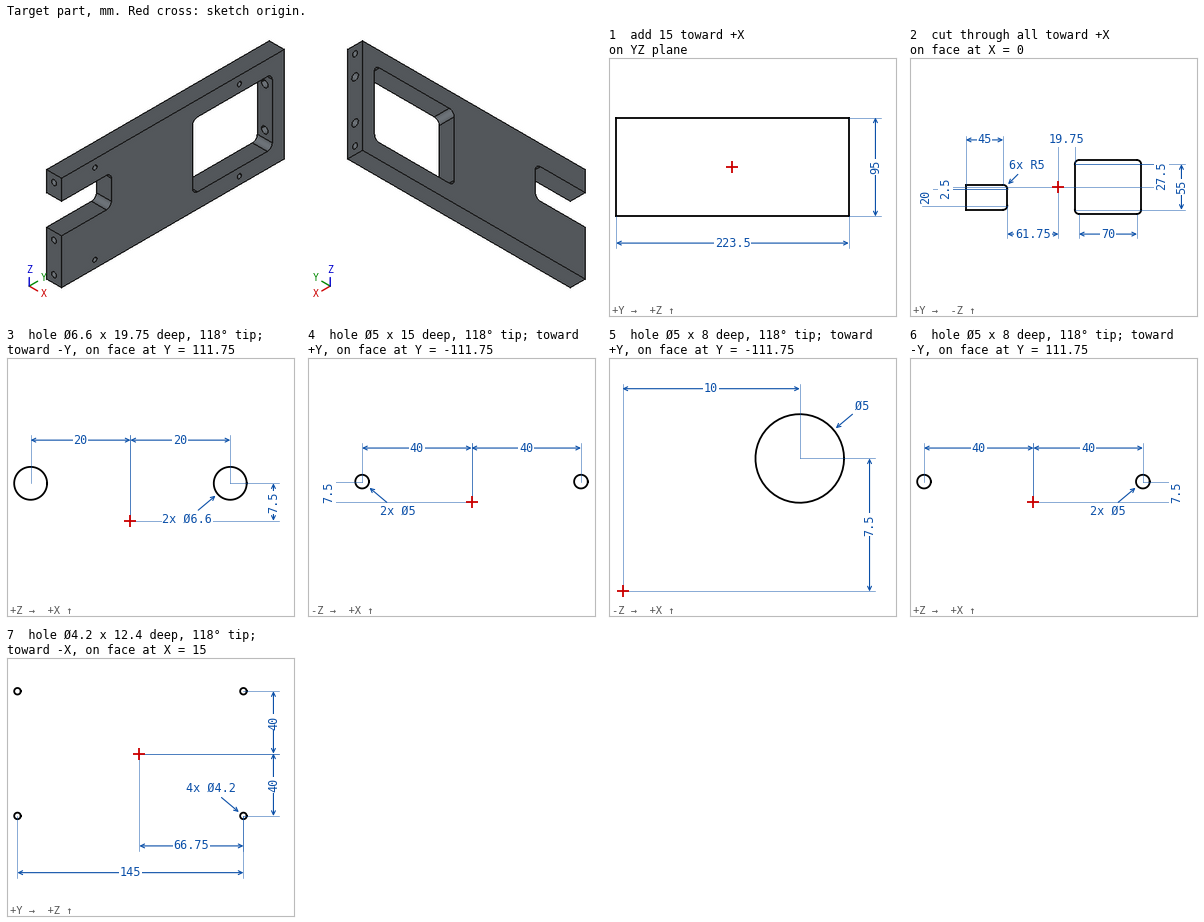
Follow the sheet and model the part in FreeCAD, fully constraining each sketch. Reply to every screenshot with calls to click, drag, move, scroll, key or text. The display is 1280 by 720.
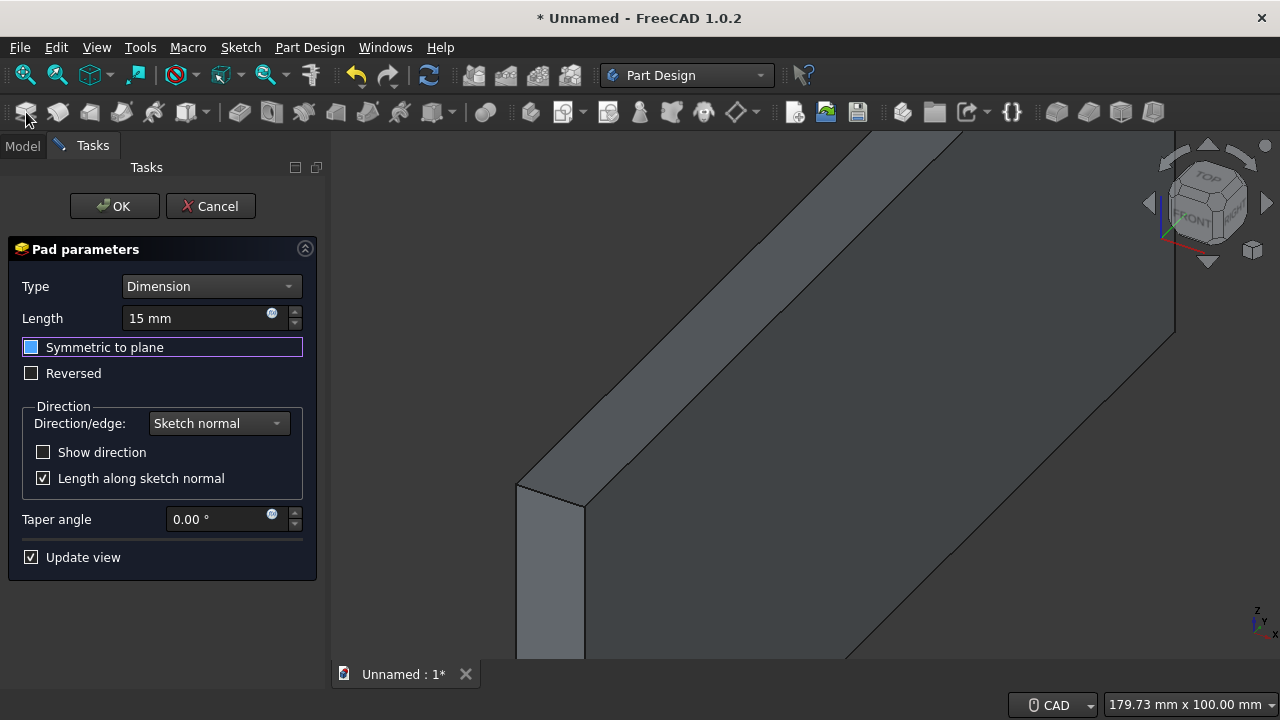
click(115, 206)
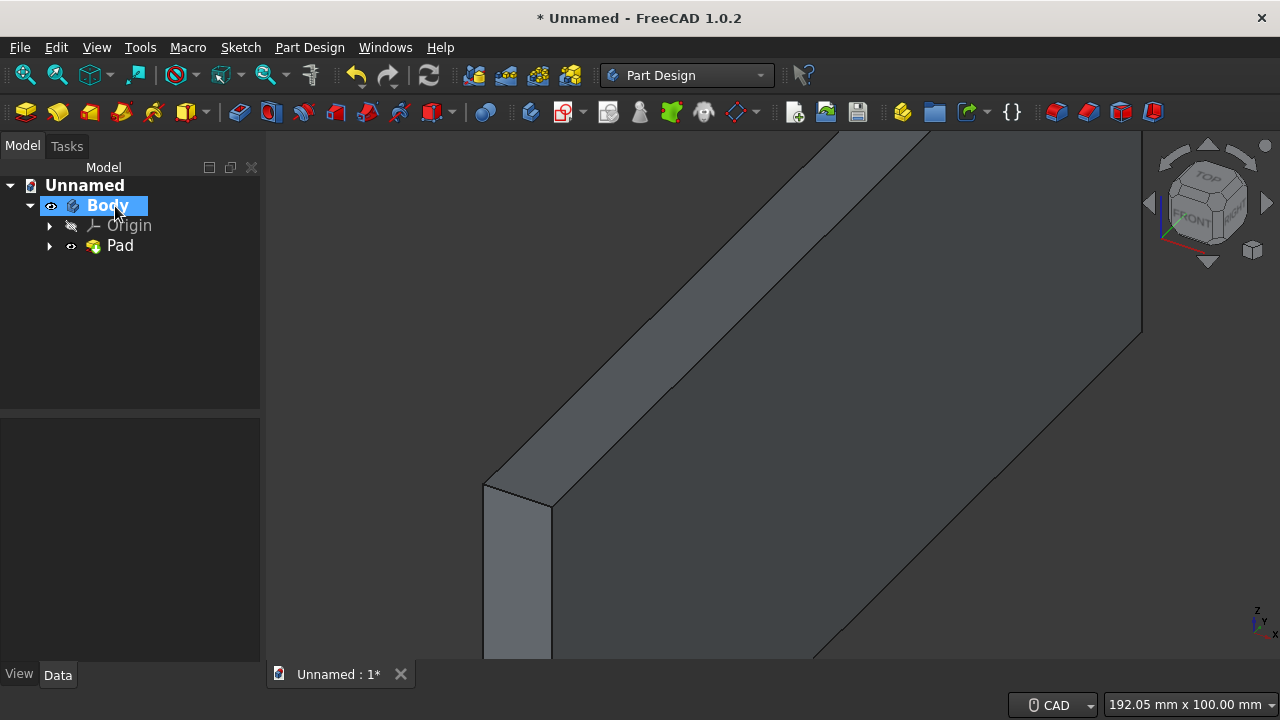
key(v)
key(f)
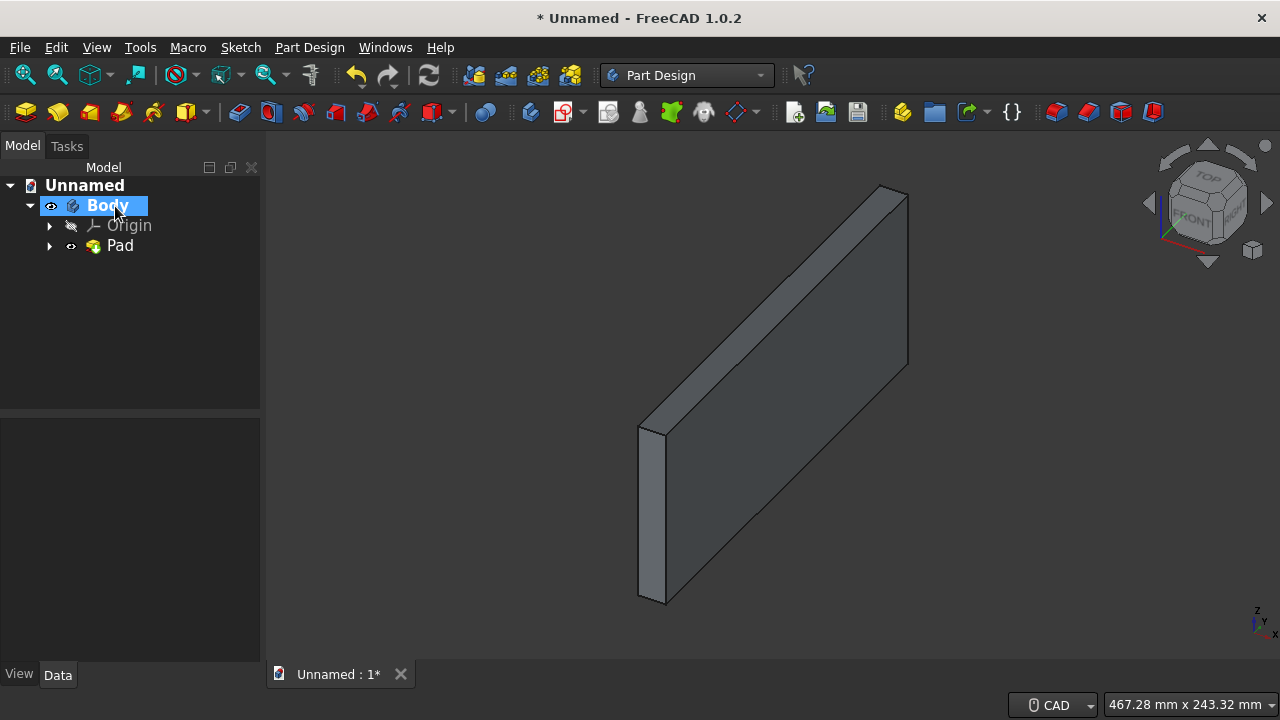
key(6)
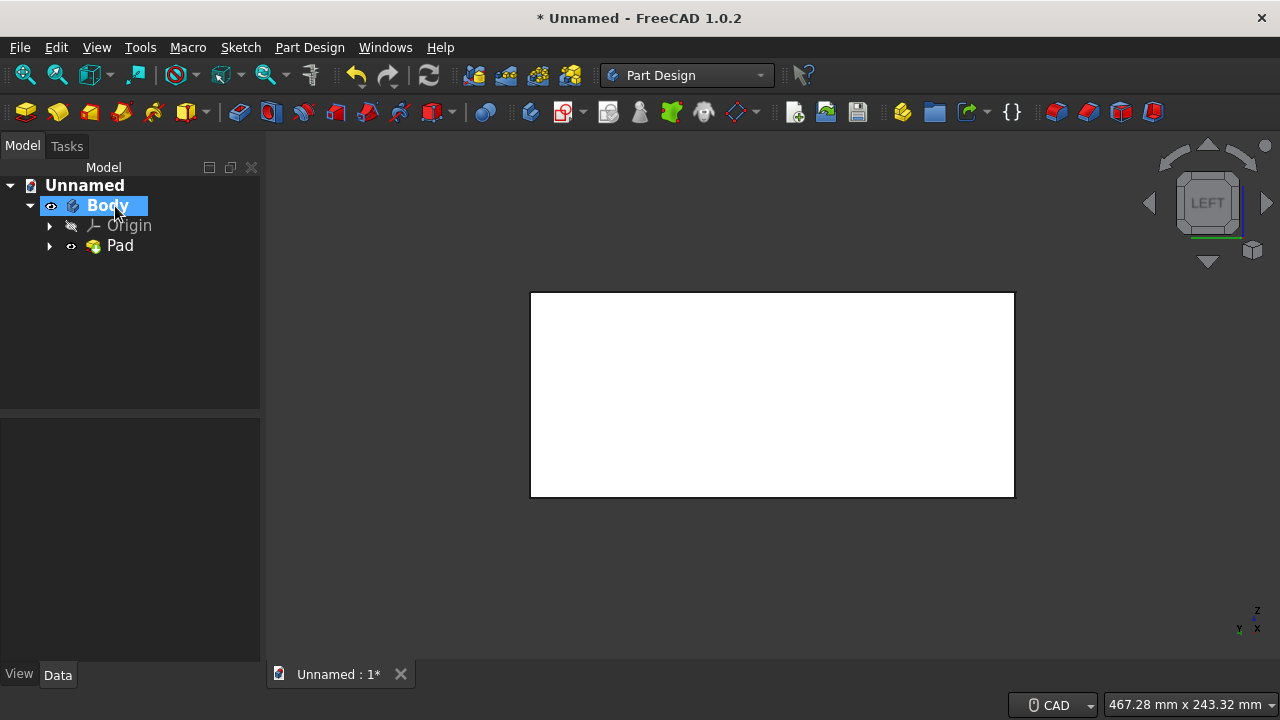
click(634, 394)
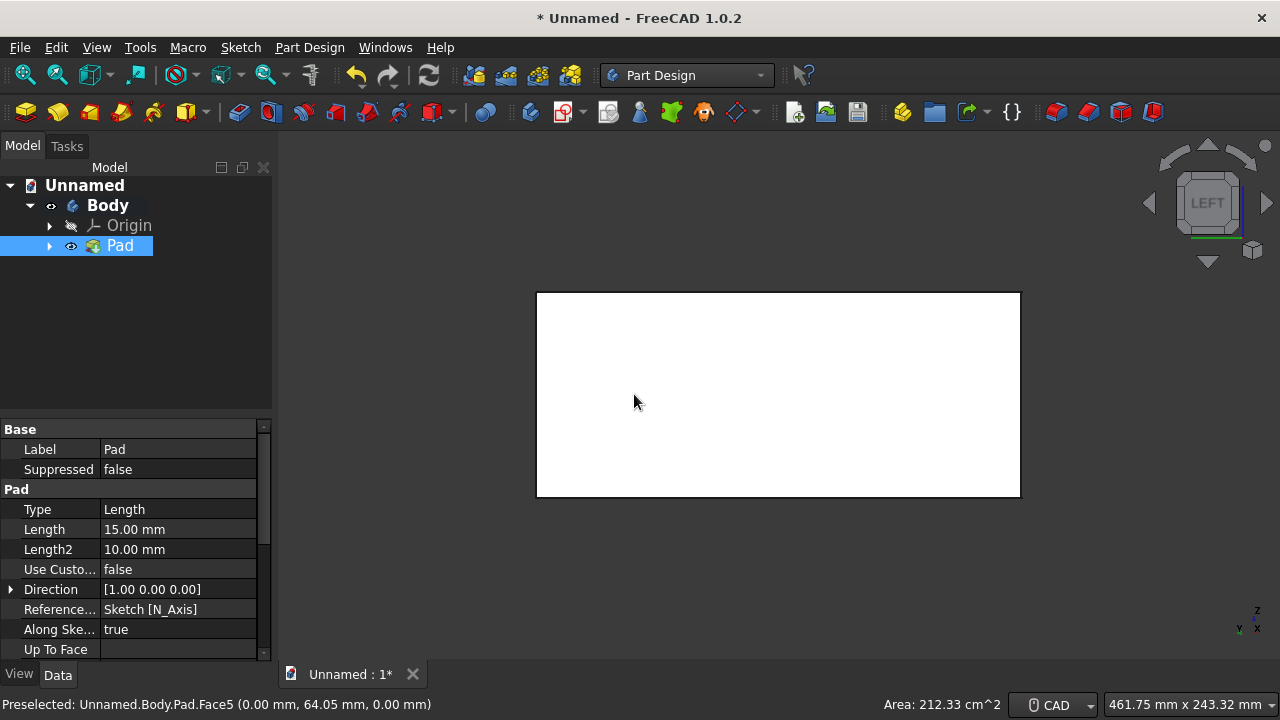
click(564, 112)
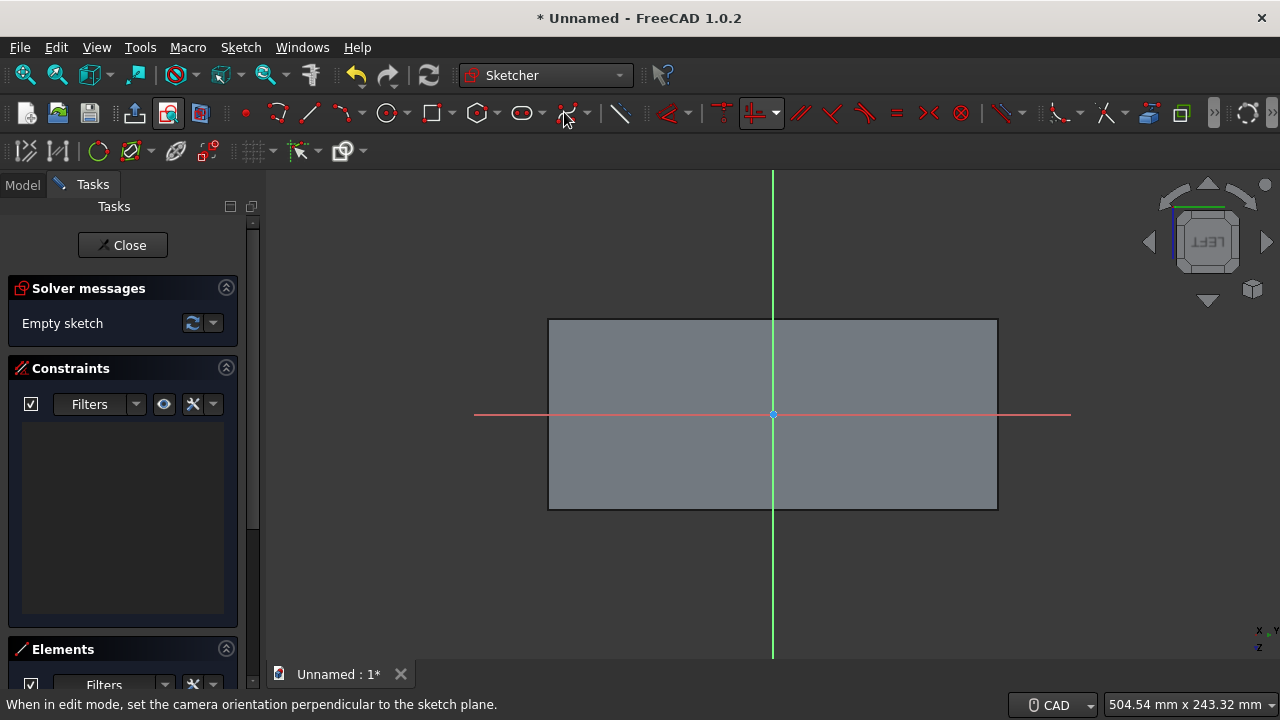
scroll(876, 414, up, 2)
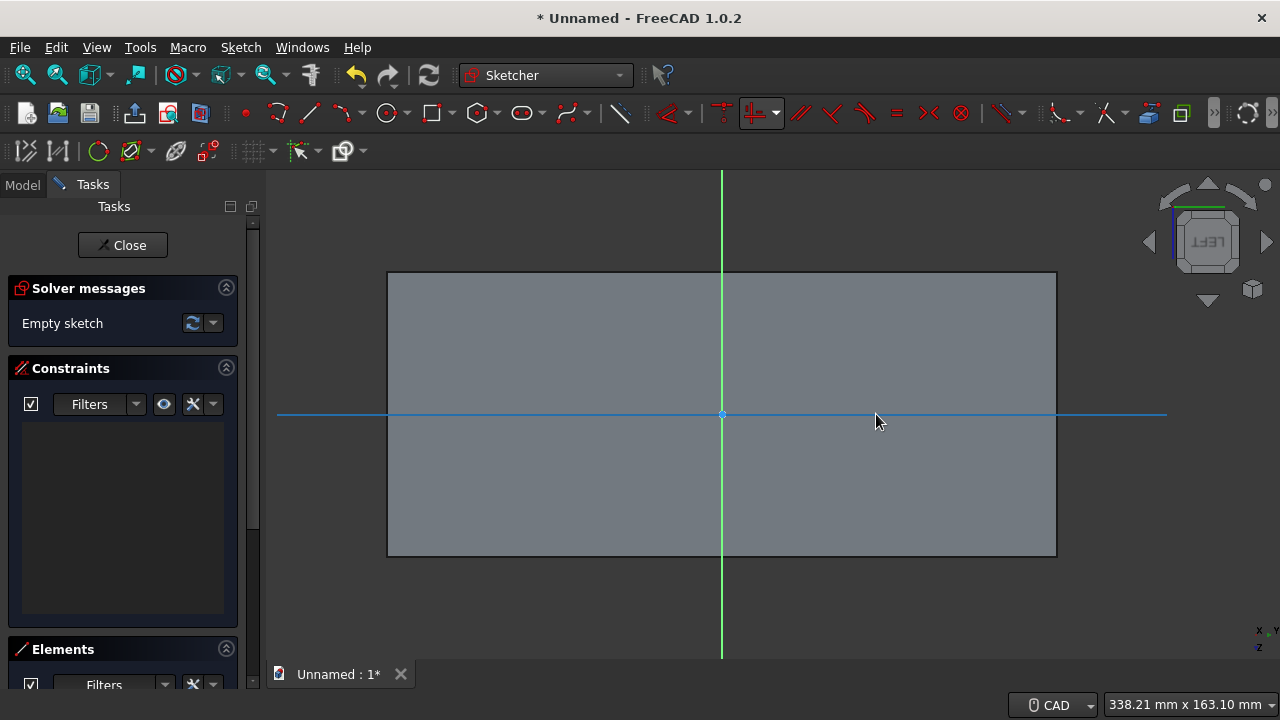
click(310, 114)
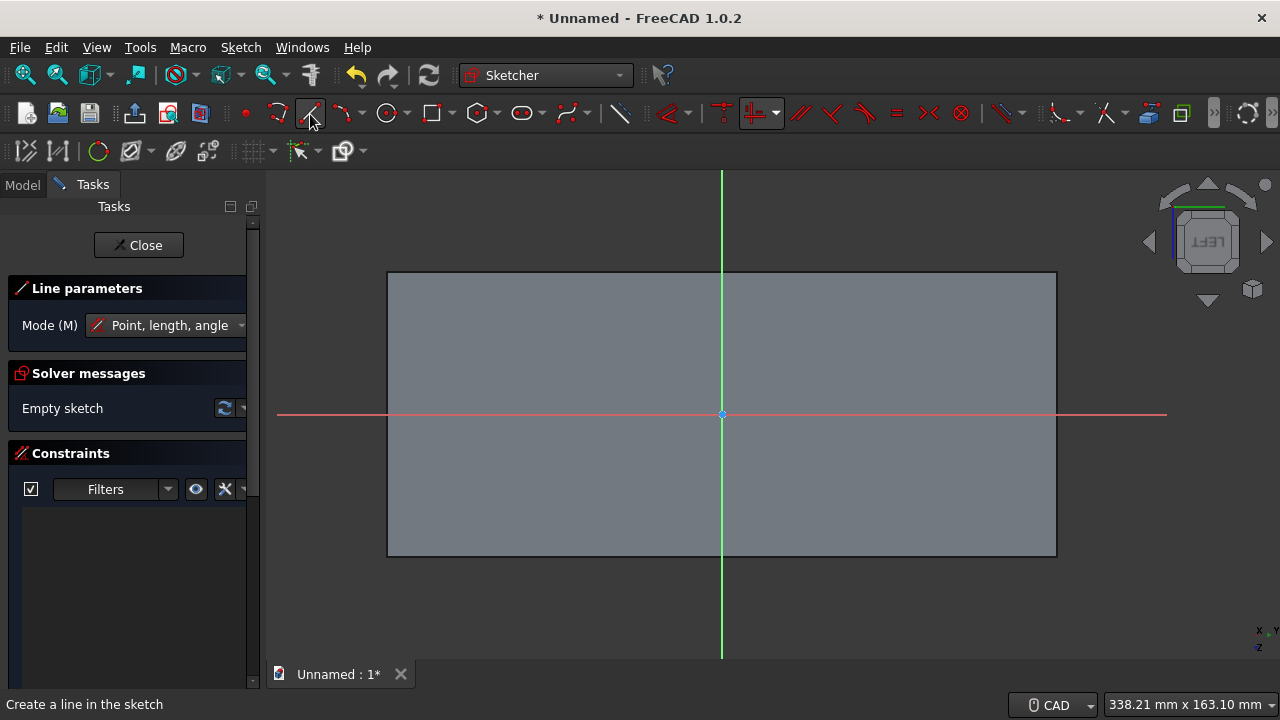
click(537, 482)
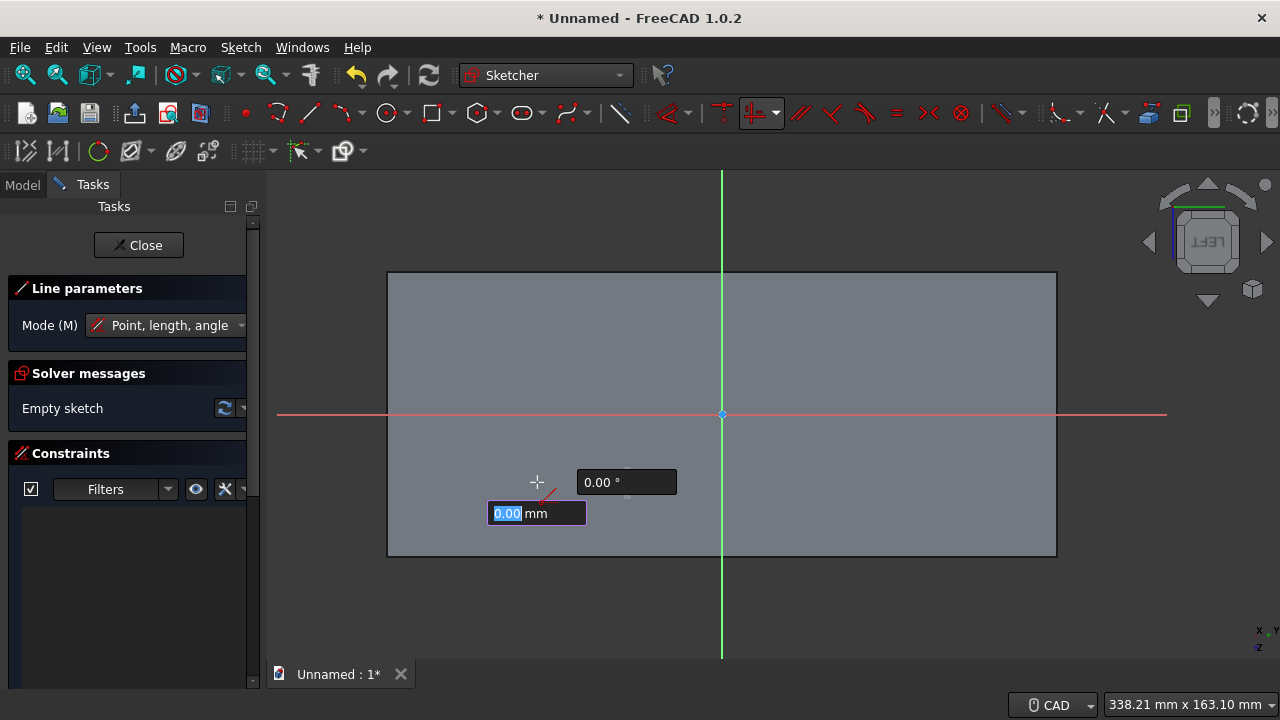
scroll(537, 422, up, 4)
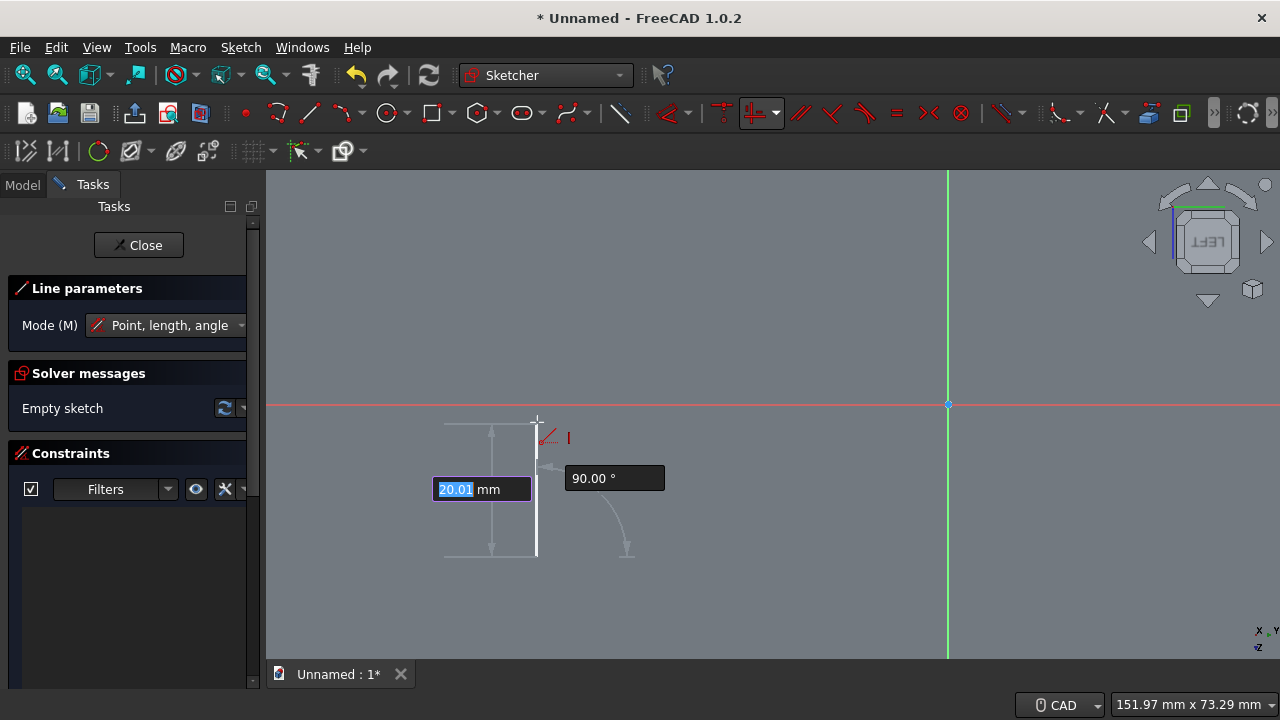
click(537, 421)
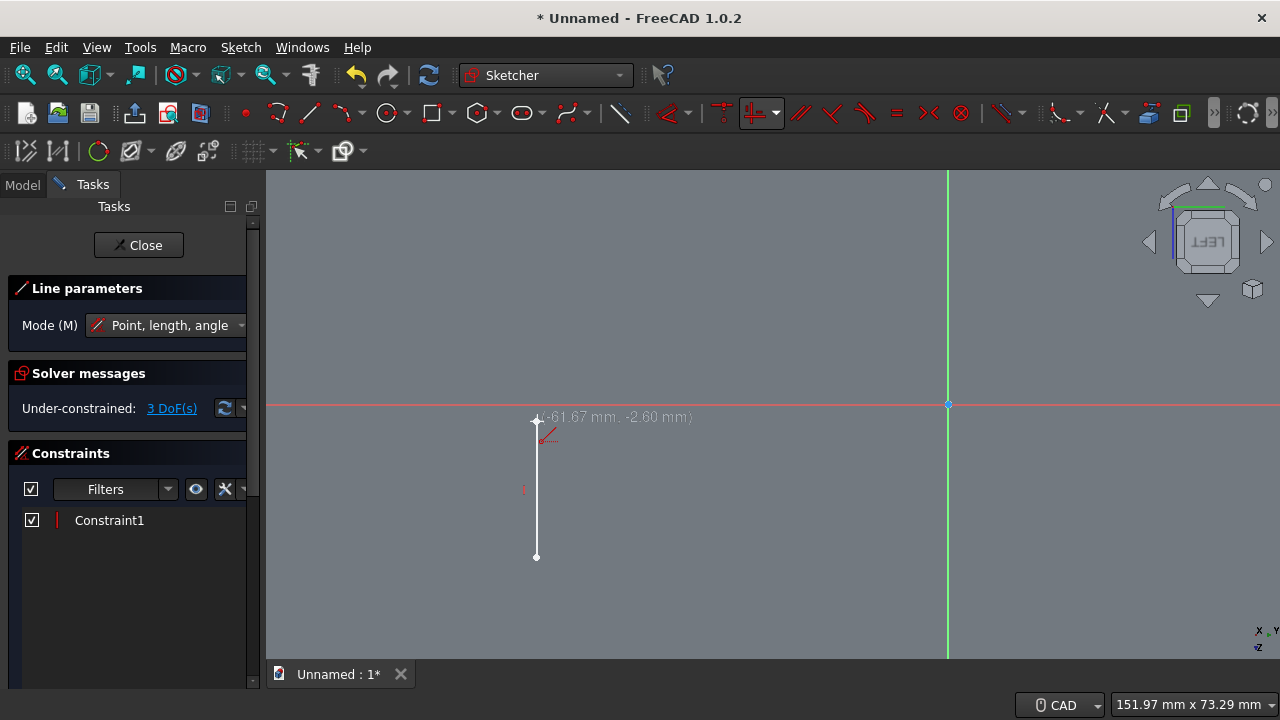
click(278, 114)